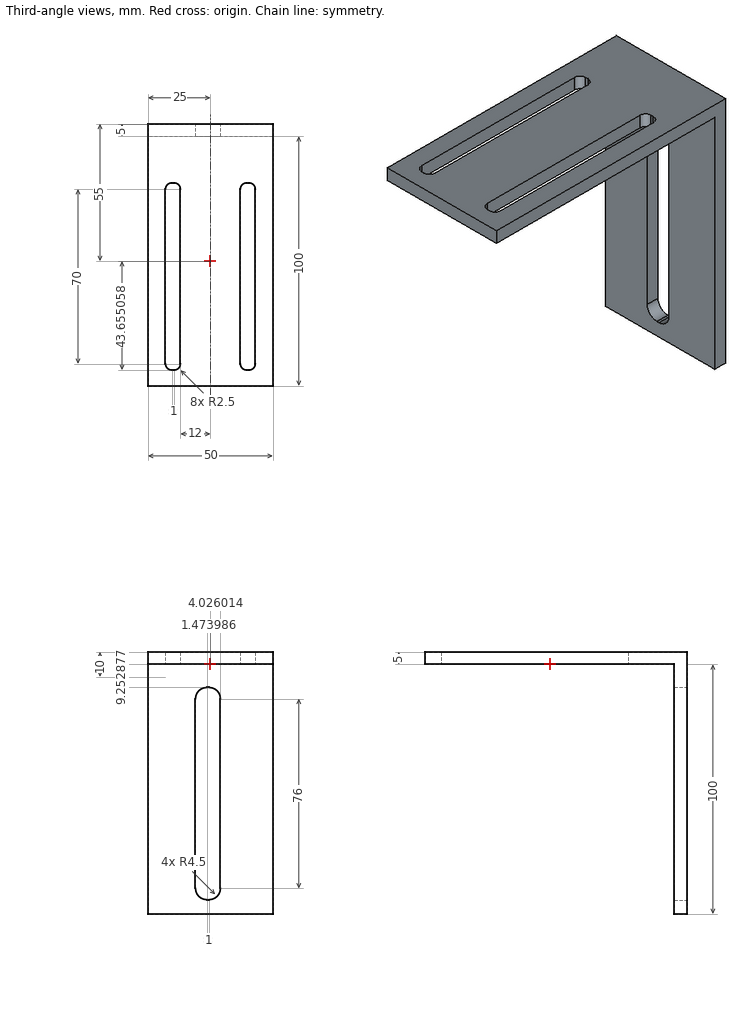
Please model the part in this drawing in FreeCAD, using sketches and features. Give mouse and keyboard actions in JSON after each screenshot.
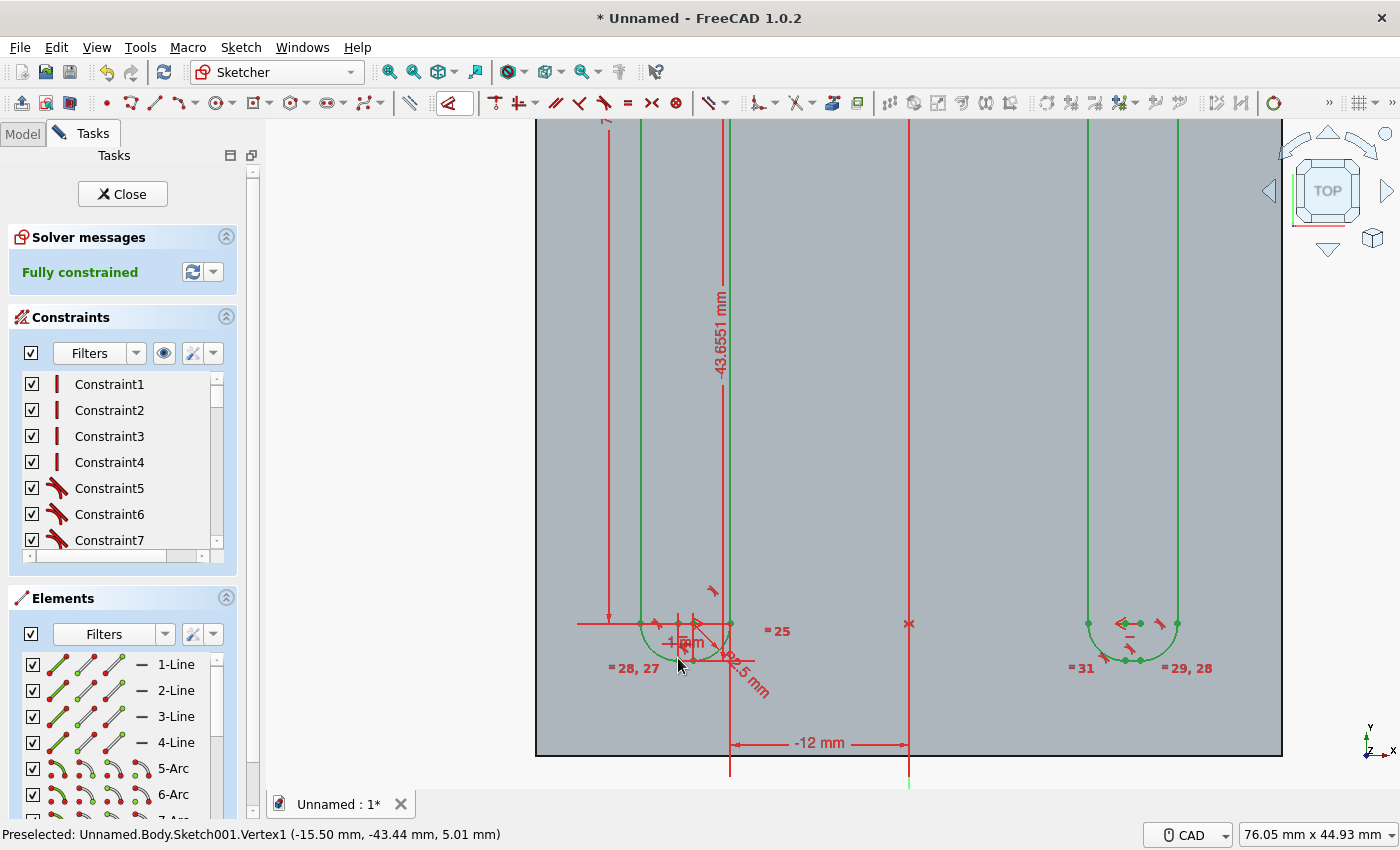
{"action": "left_click", "coordinate": [123, 194]}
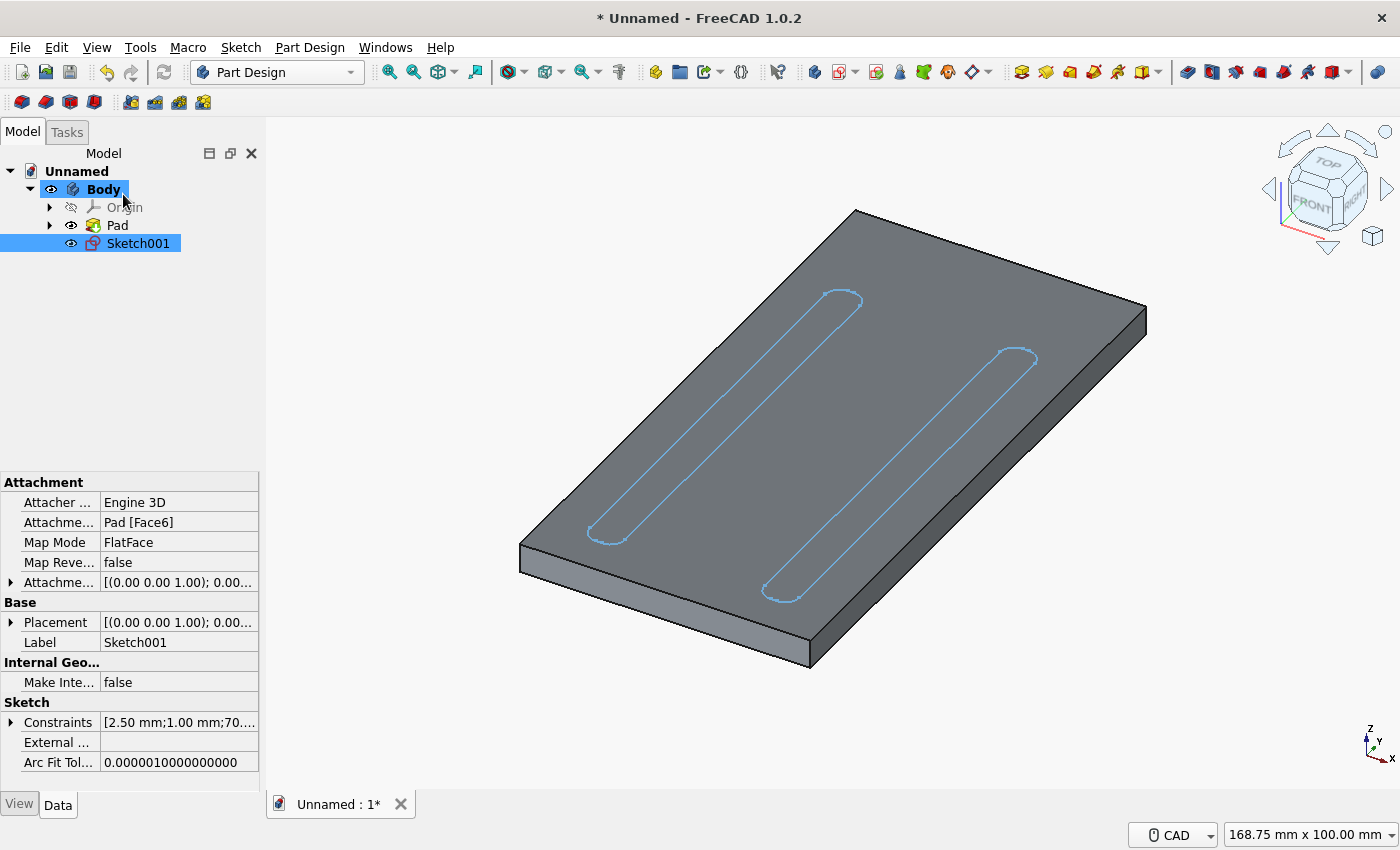
{"action": "left_click", "coordinate": [1188, 72]}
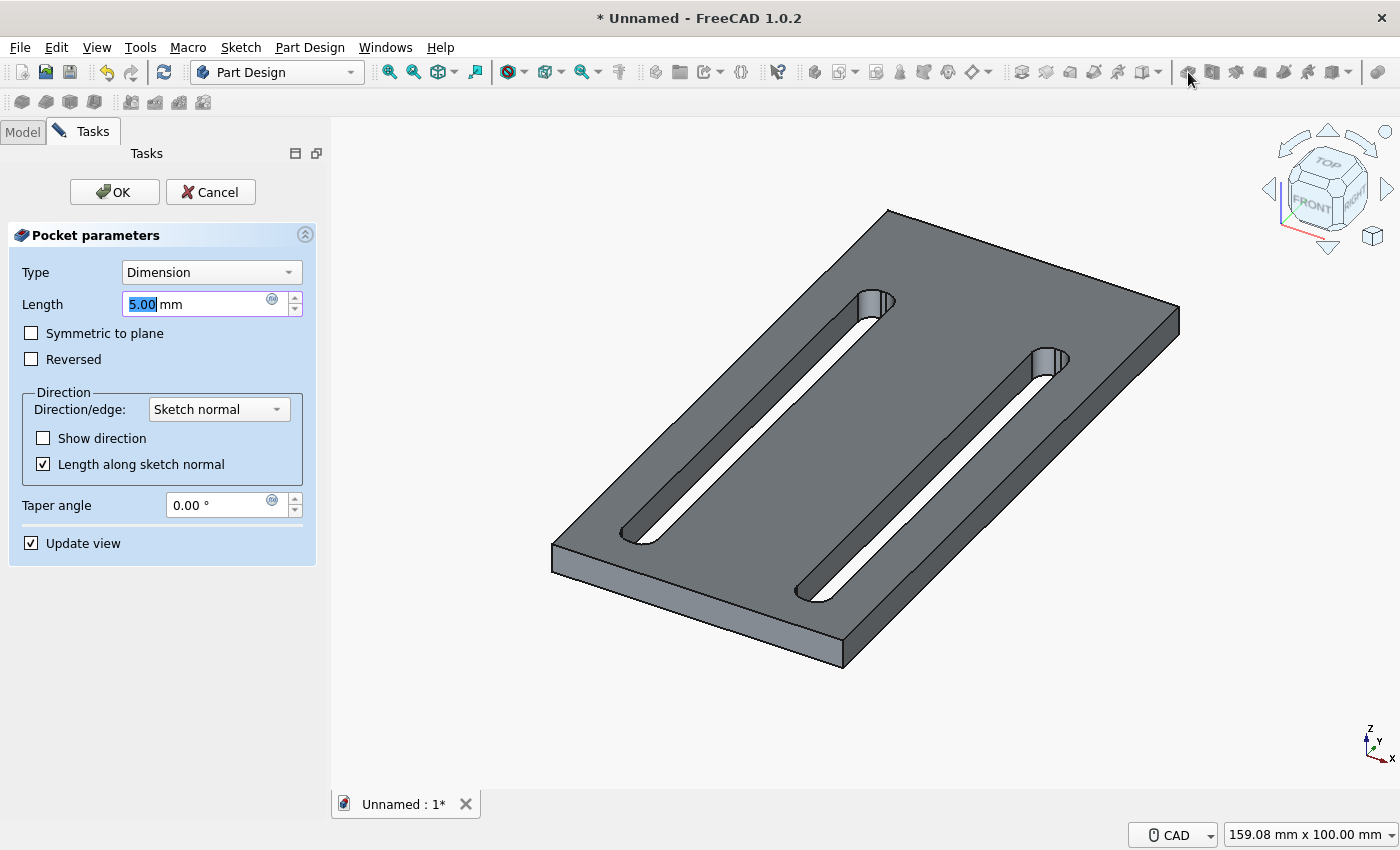
{"action": "type", "text": "10"}
{"action": "key", "text": "Tab"}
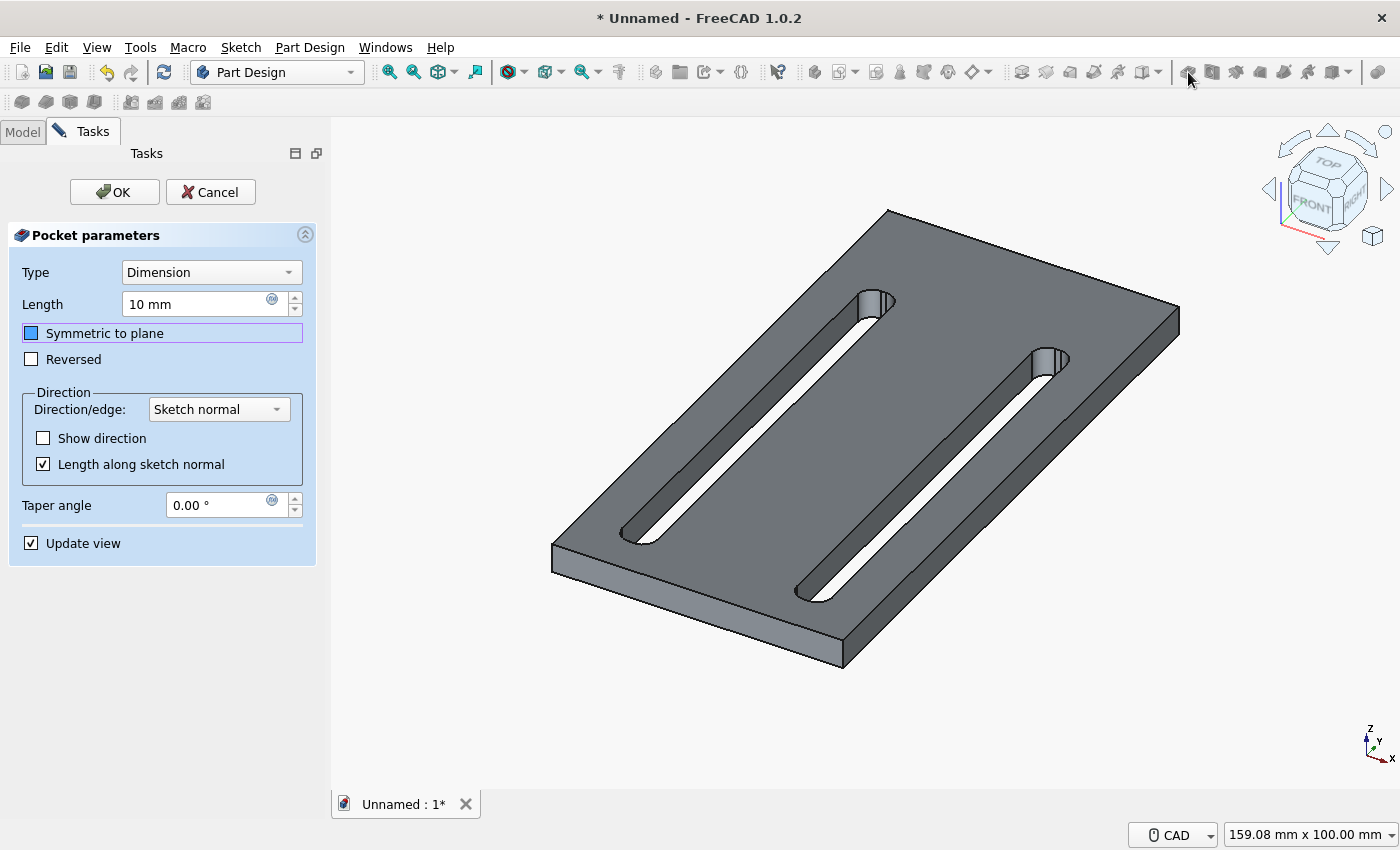
{"action": "left_click", "coordinate": [115, 192]}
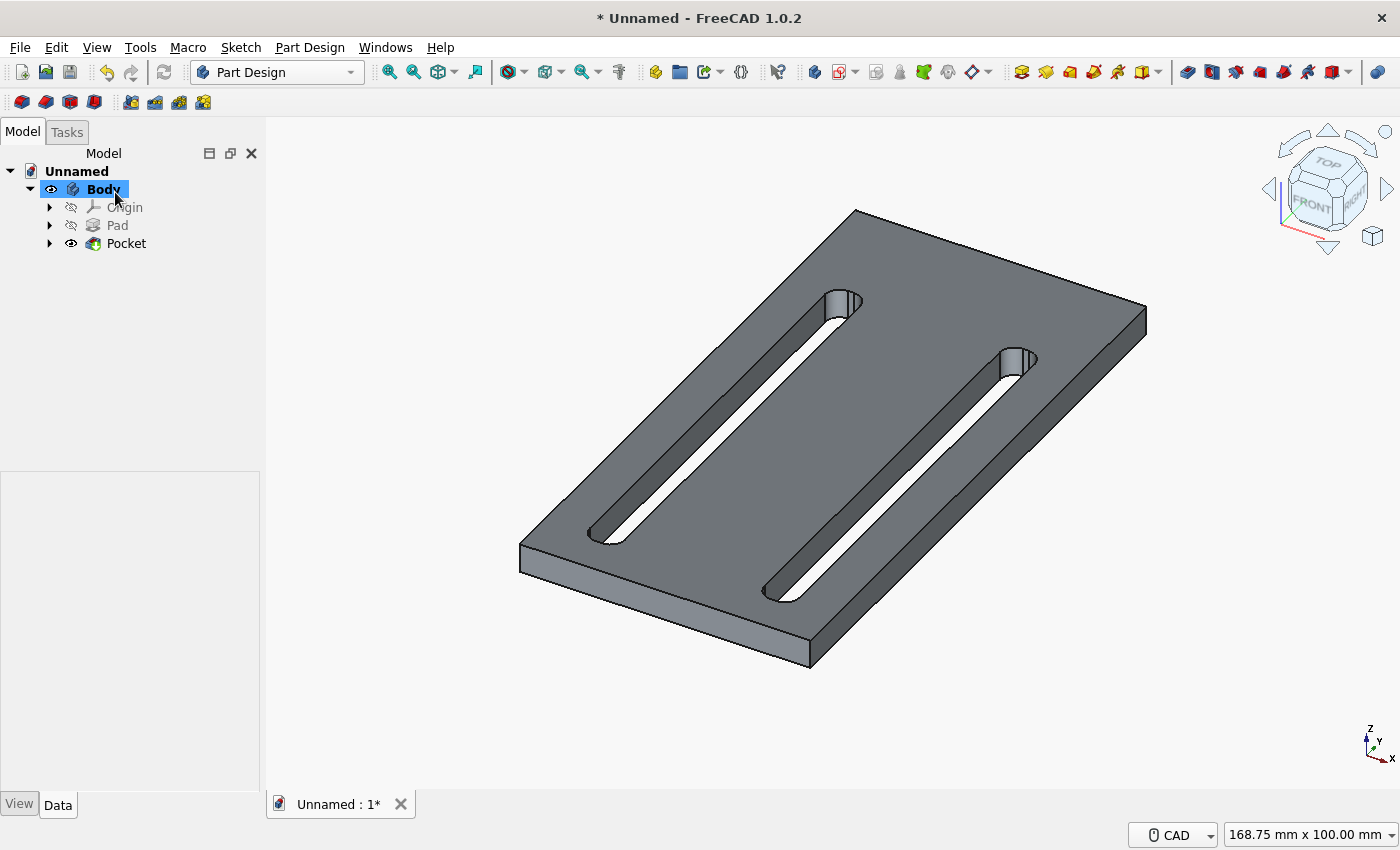
{"action": "left_click", "coordinate": [840, 72]}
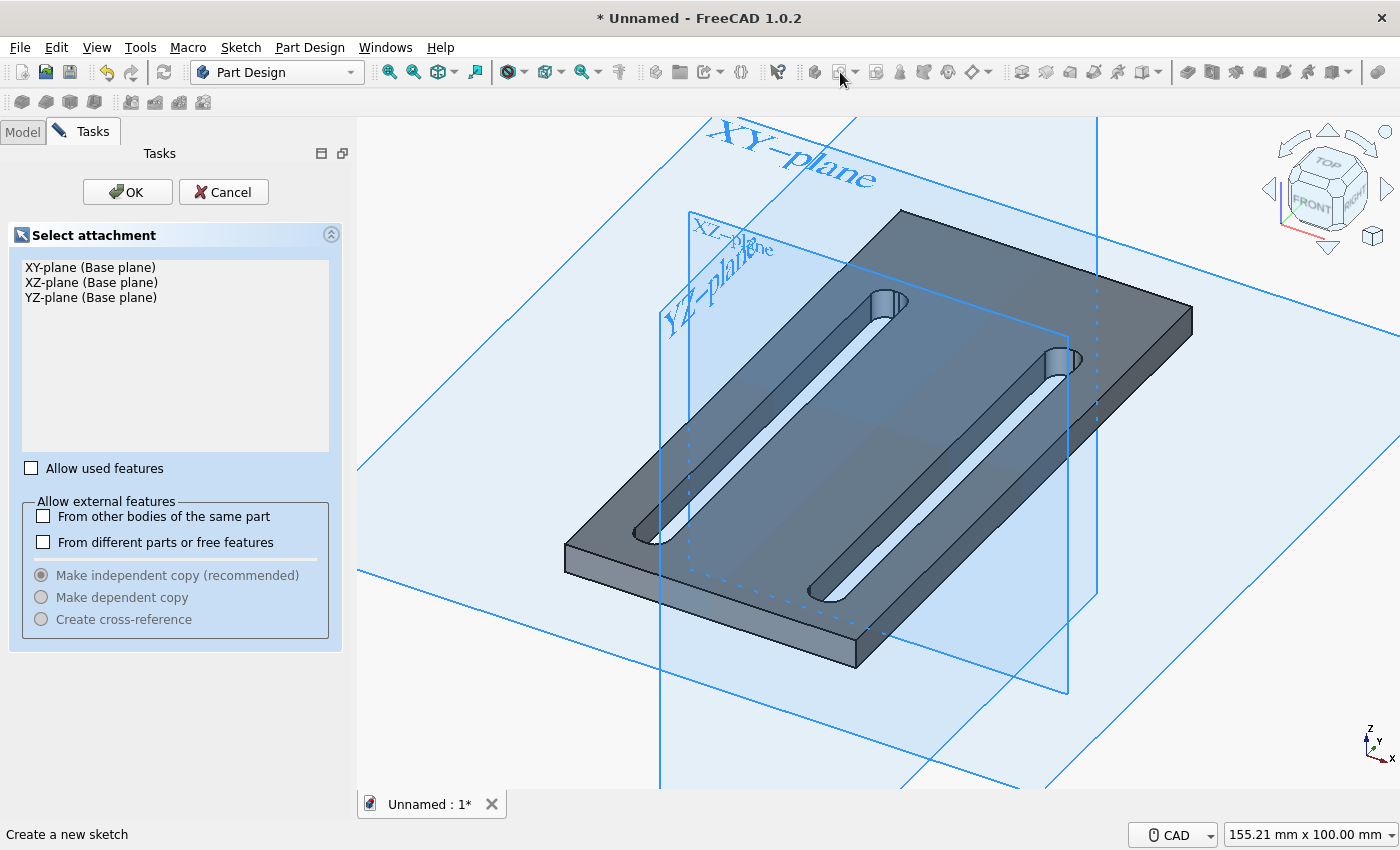
{"action": "left_click", "coordinate": [82, 268]}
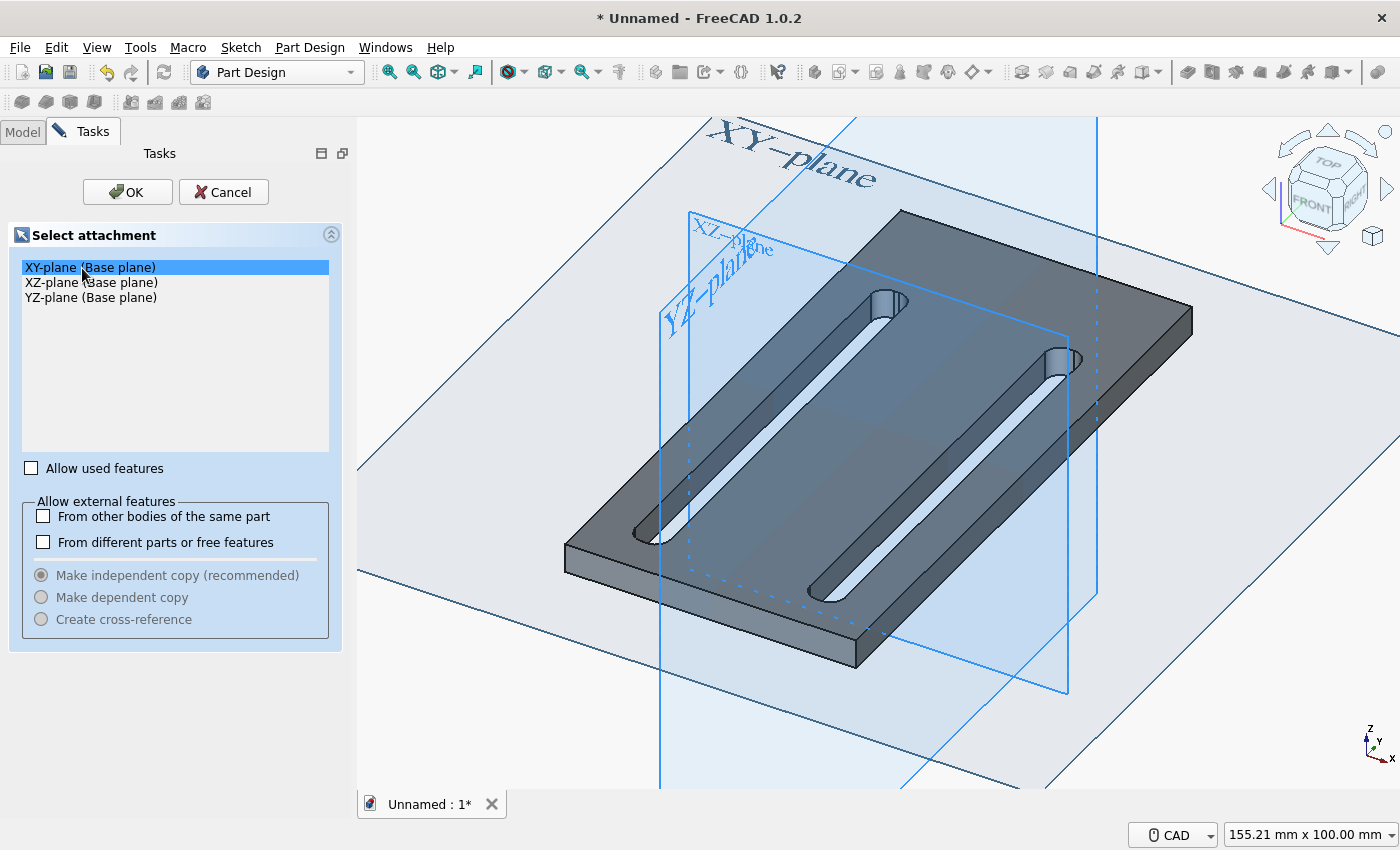
{"action": "left_click", "coordinate": [128, 192]}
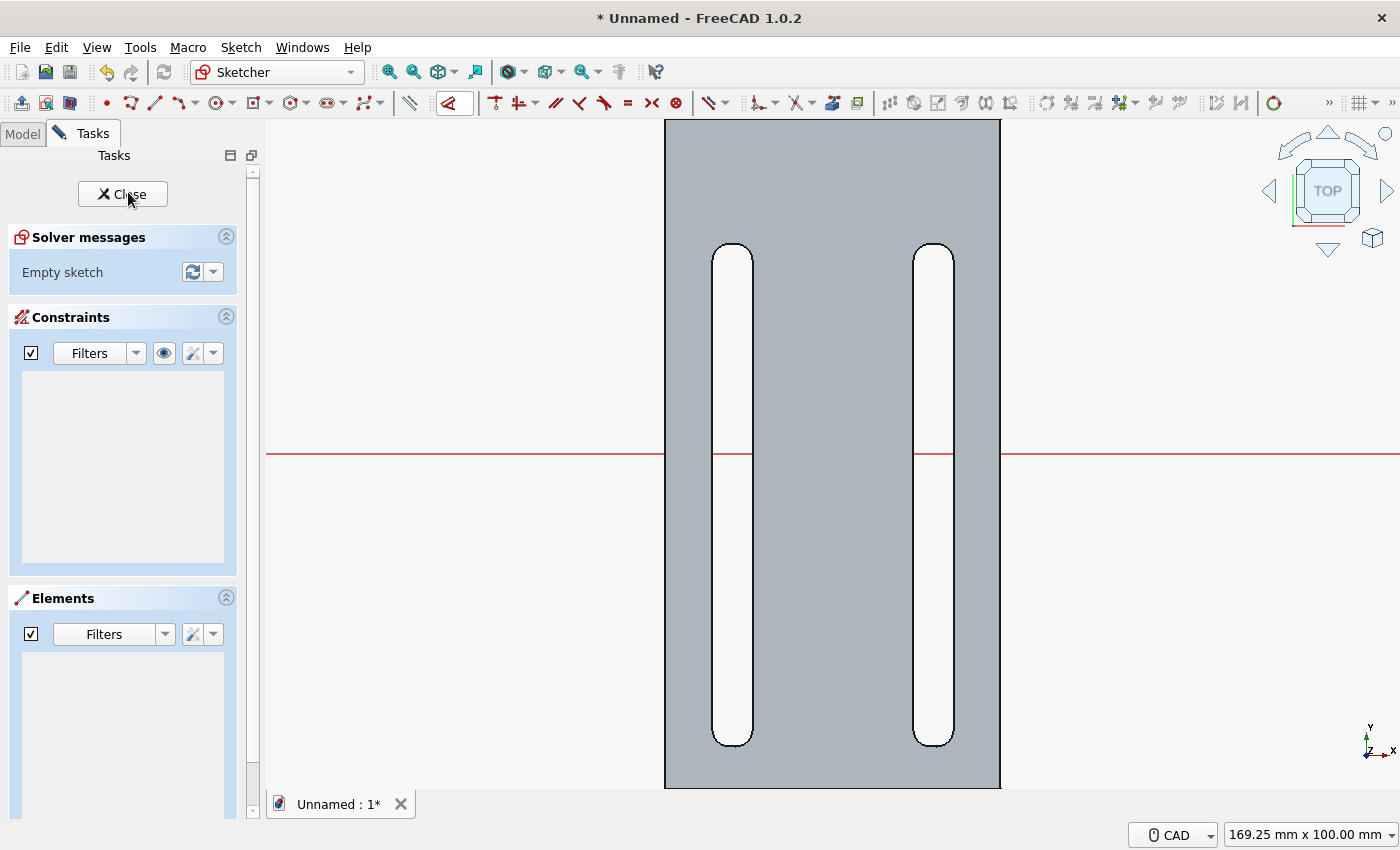
{"action": "key", "text": "q s"}